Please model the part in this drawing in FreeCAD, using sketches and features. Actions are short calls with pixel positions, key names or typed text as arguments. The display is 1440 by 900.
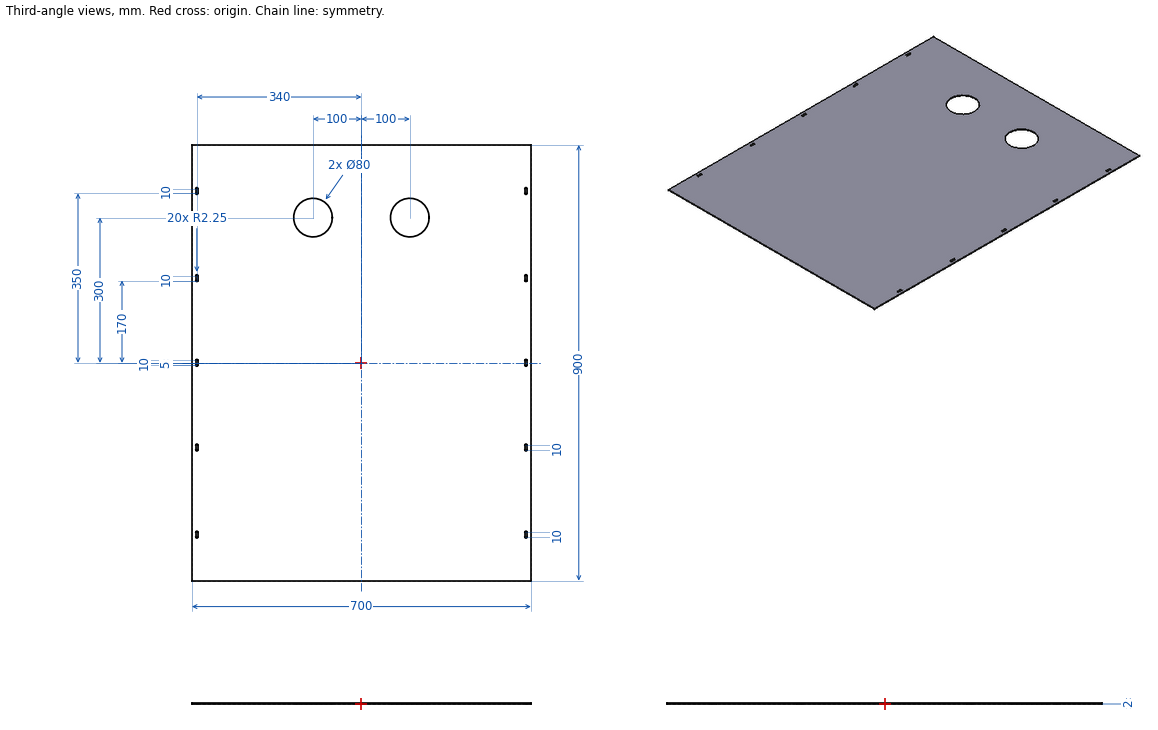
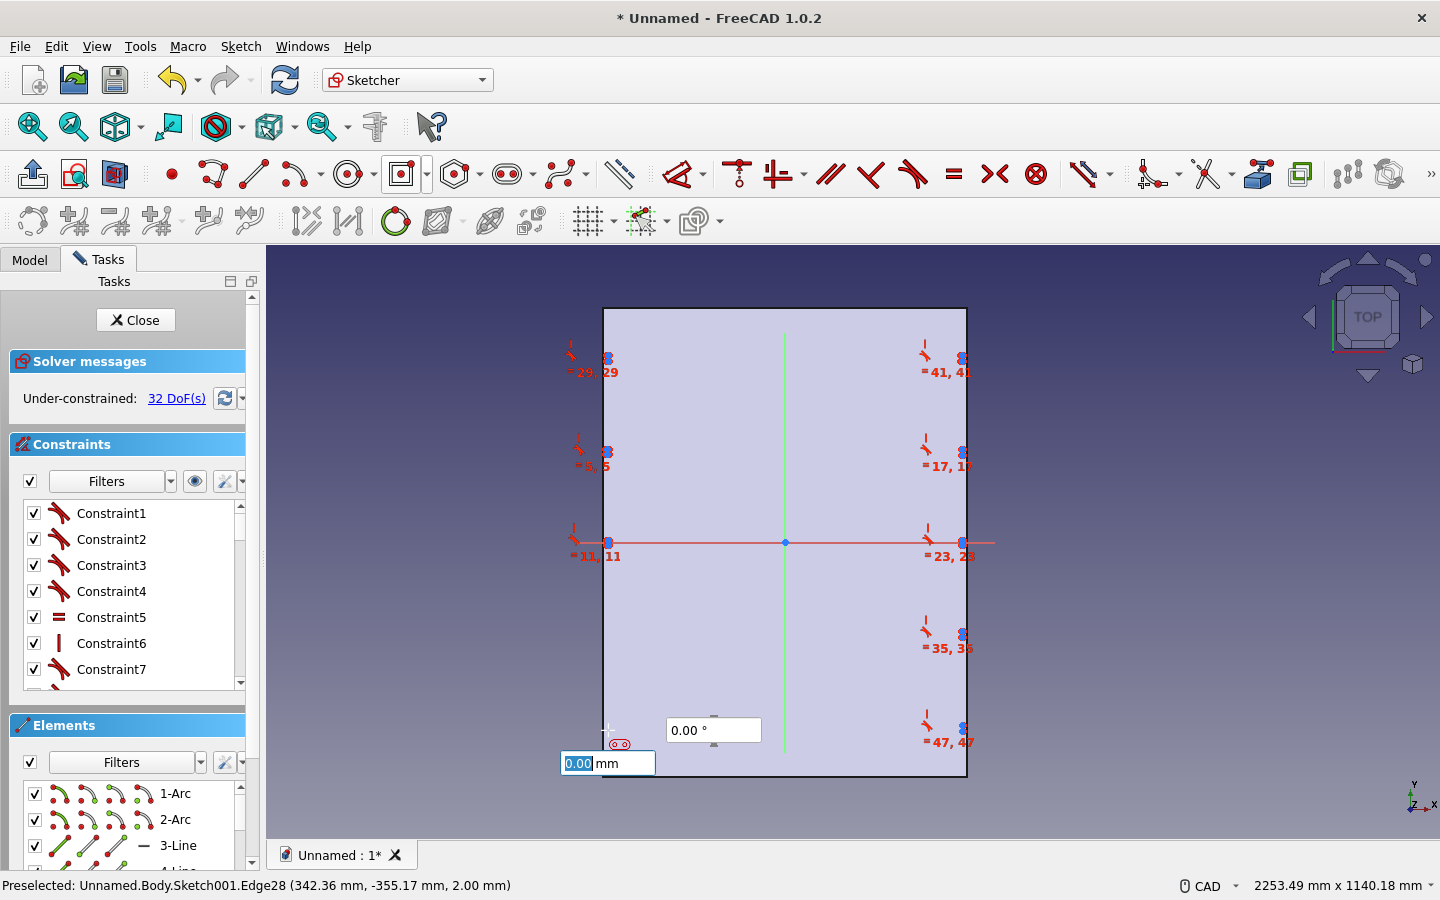
scroll(608, 725, up, 6)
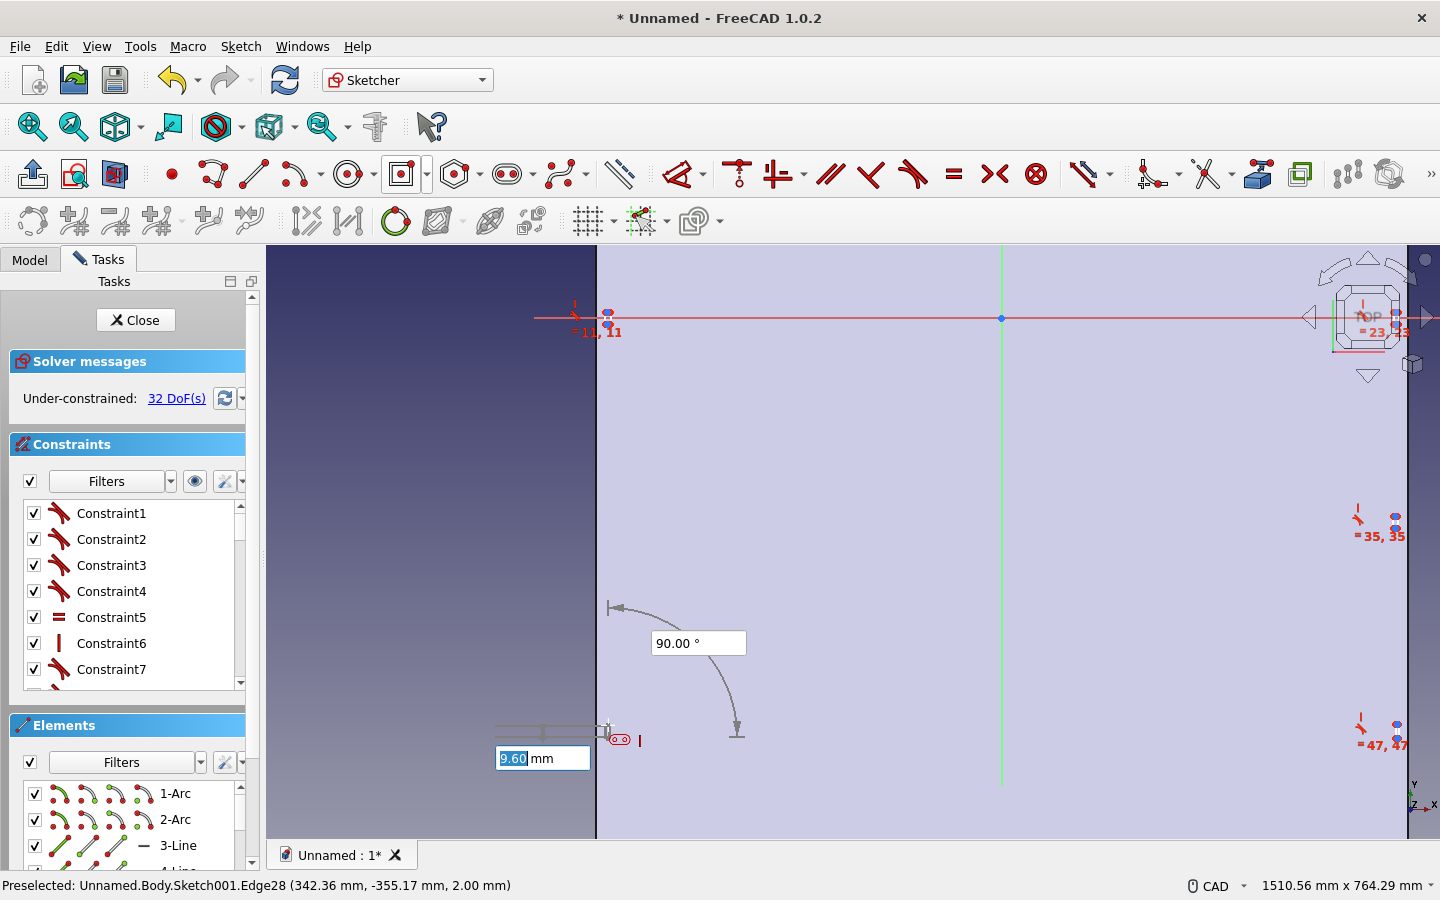
click(607, 724)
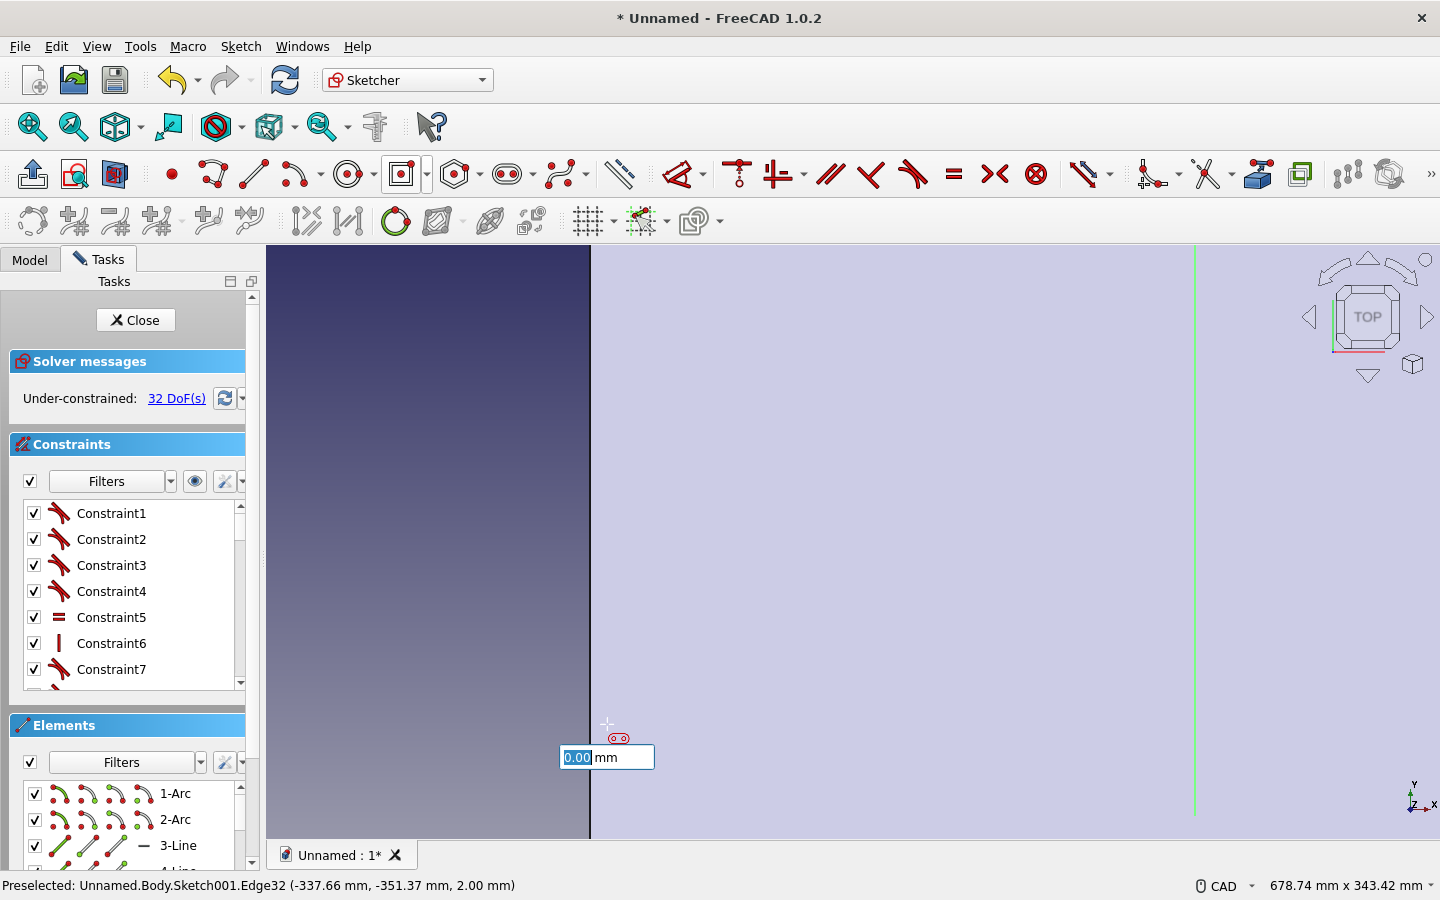
scroll(603, 732, up, 8)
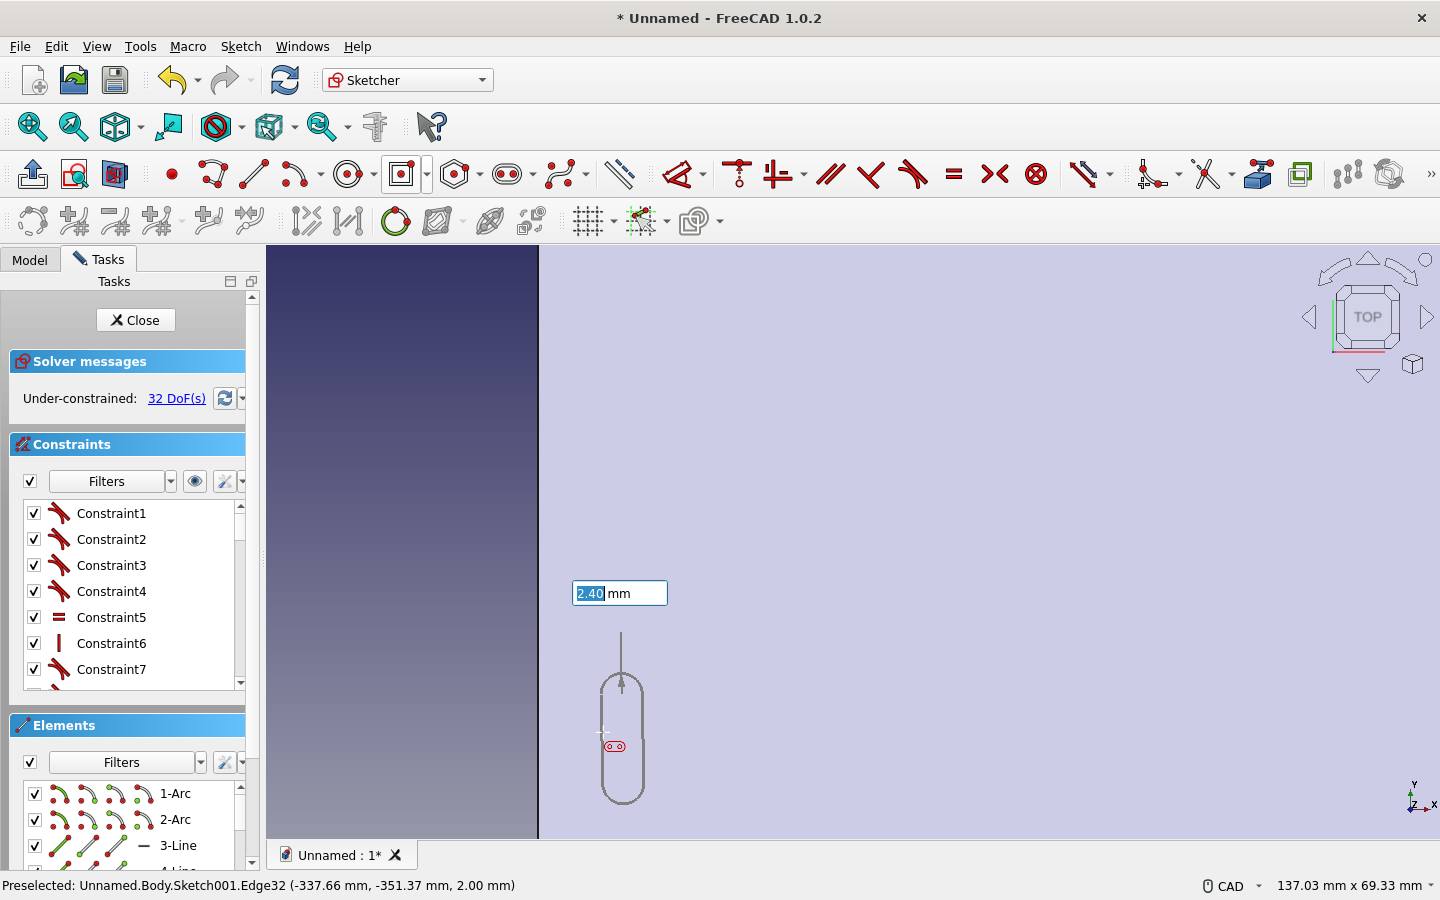
click(604, 730)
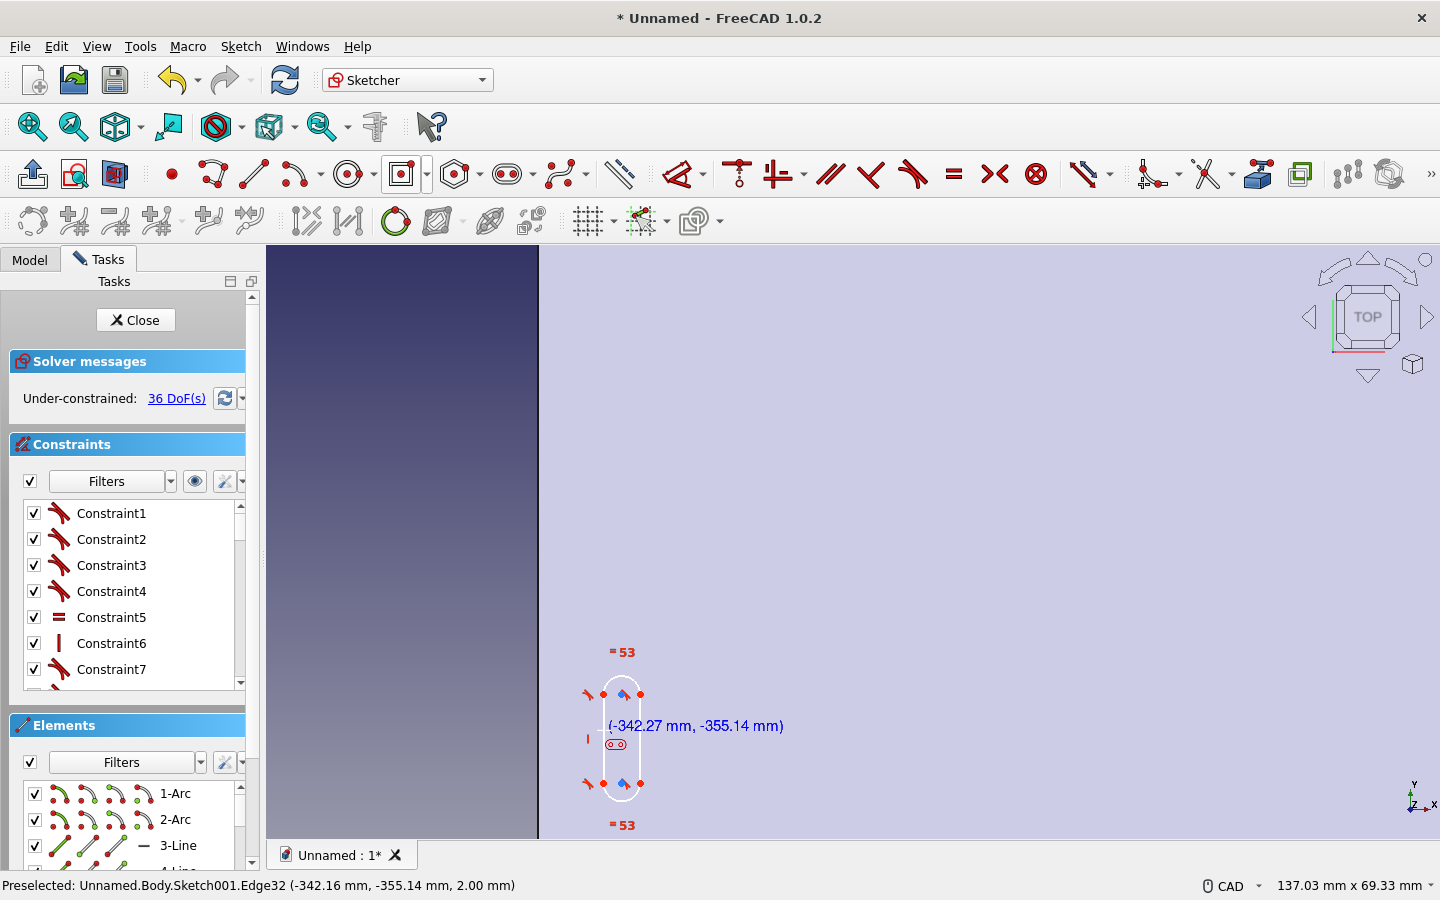
scroll(606, 727, down, 14)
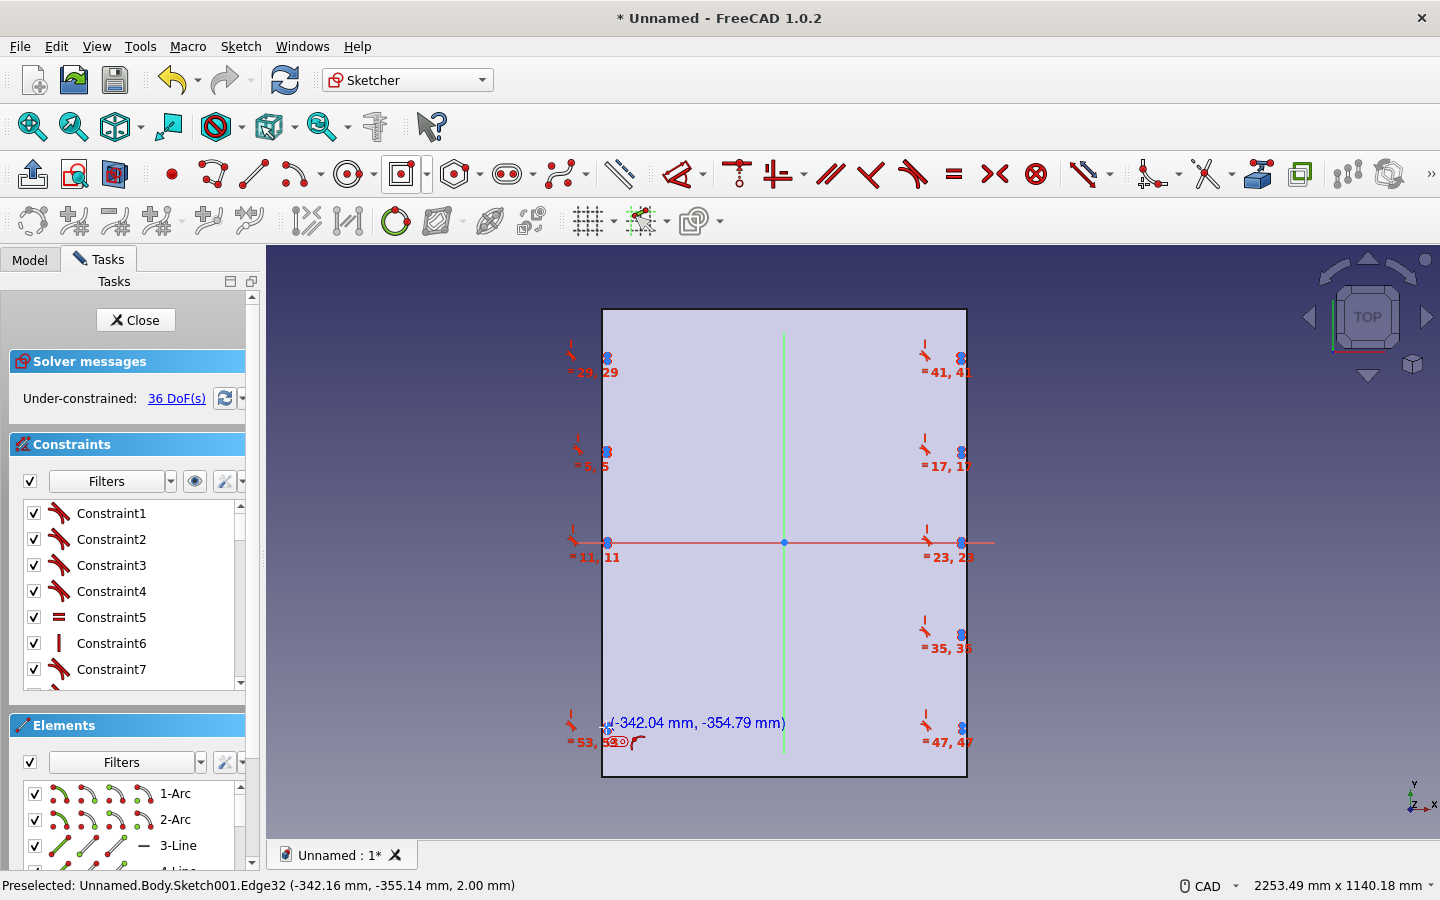
scroll(607, 637, up, 15)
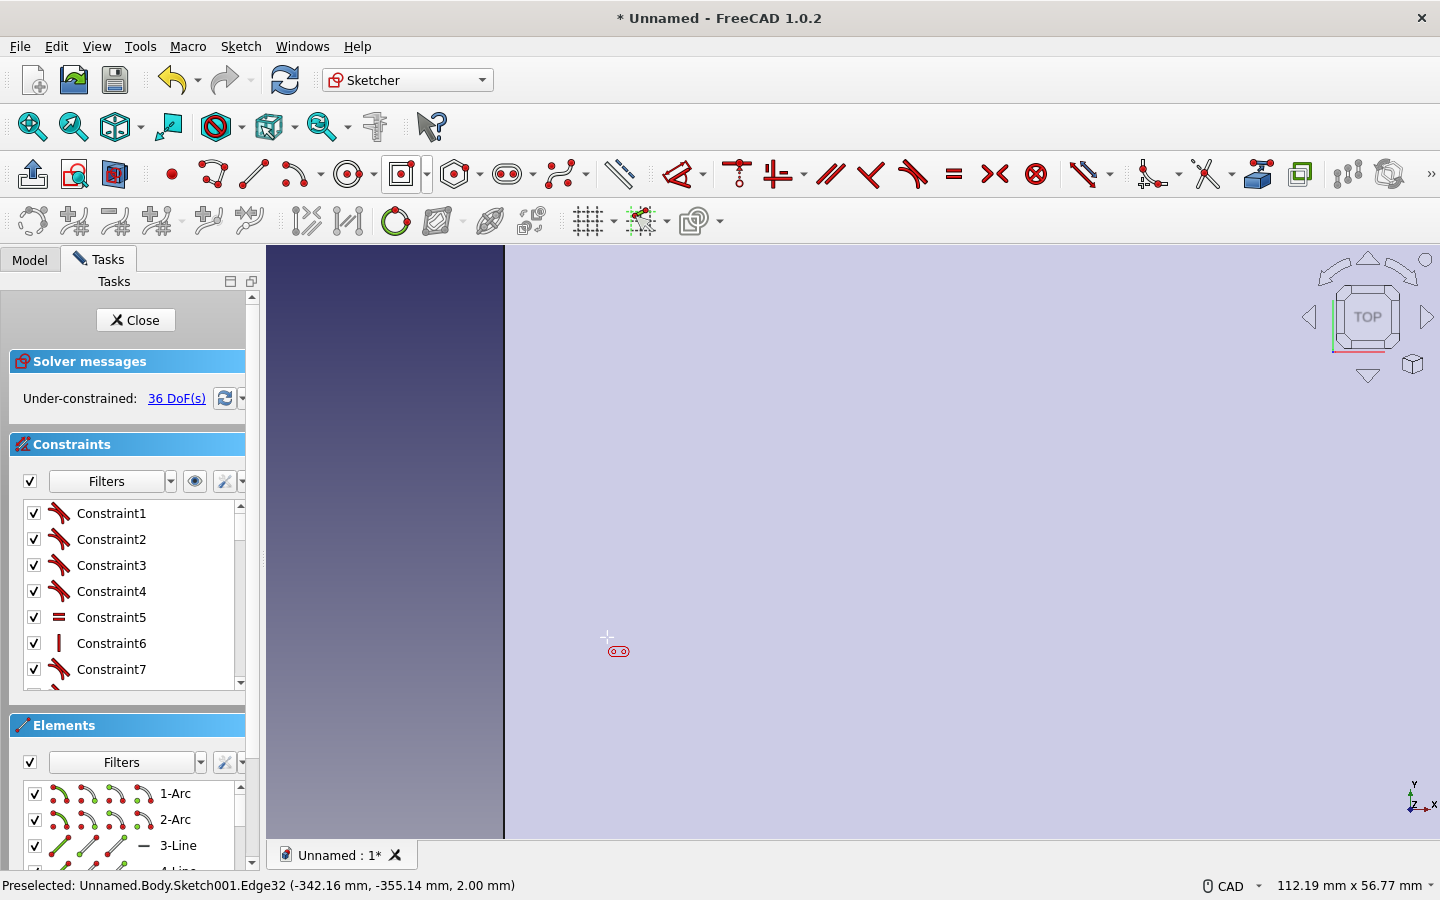
scroll(607, 637, down, 15)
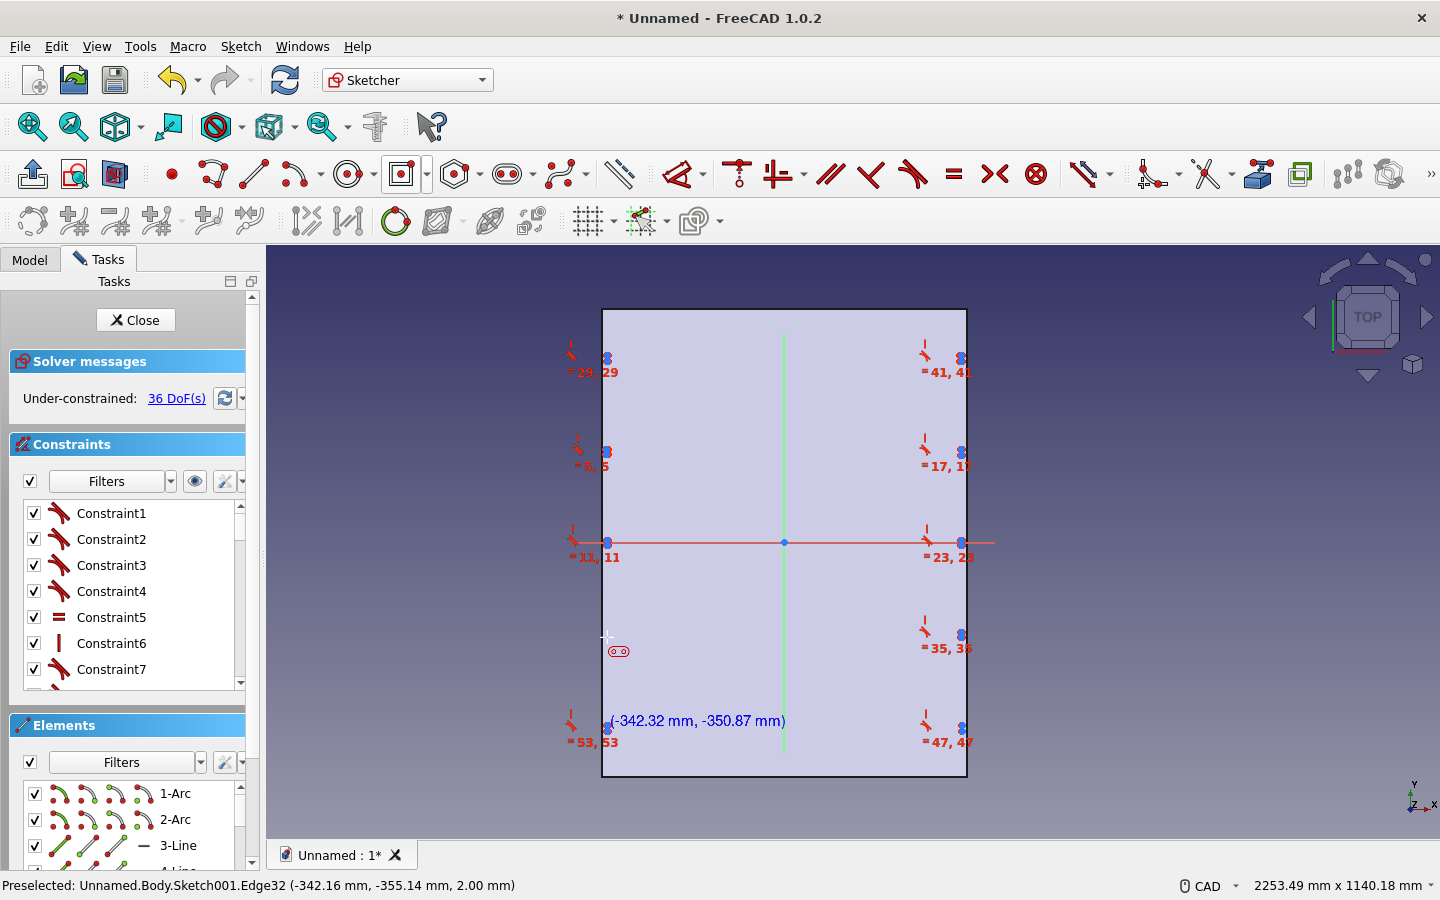
click(607, 637)